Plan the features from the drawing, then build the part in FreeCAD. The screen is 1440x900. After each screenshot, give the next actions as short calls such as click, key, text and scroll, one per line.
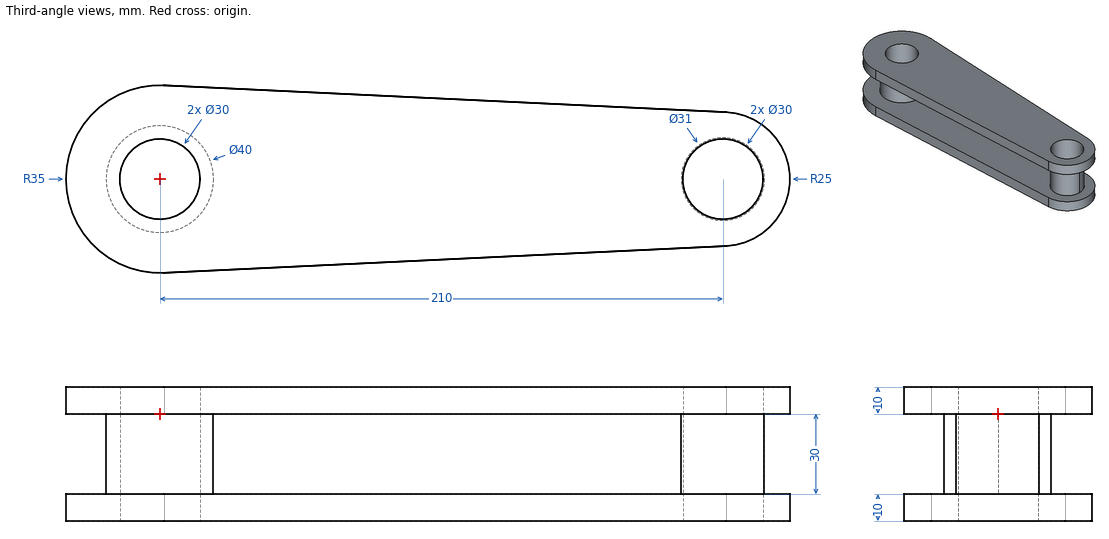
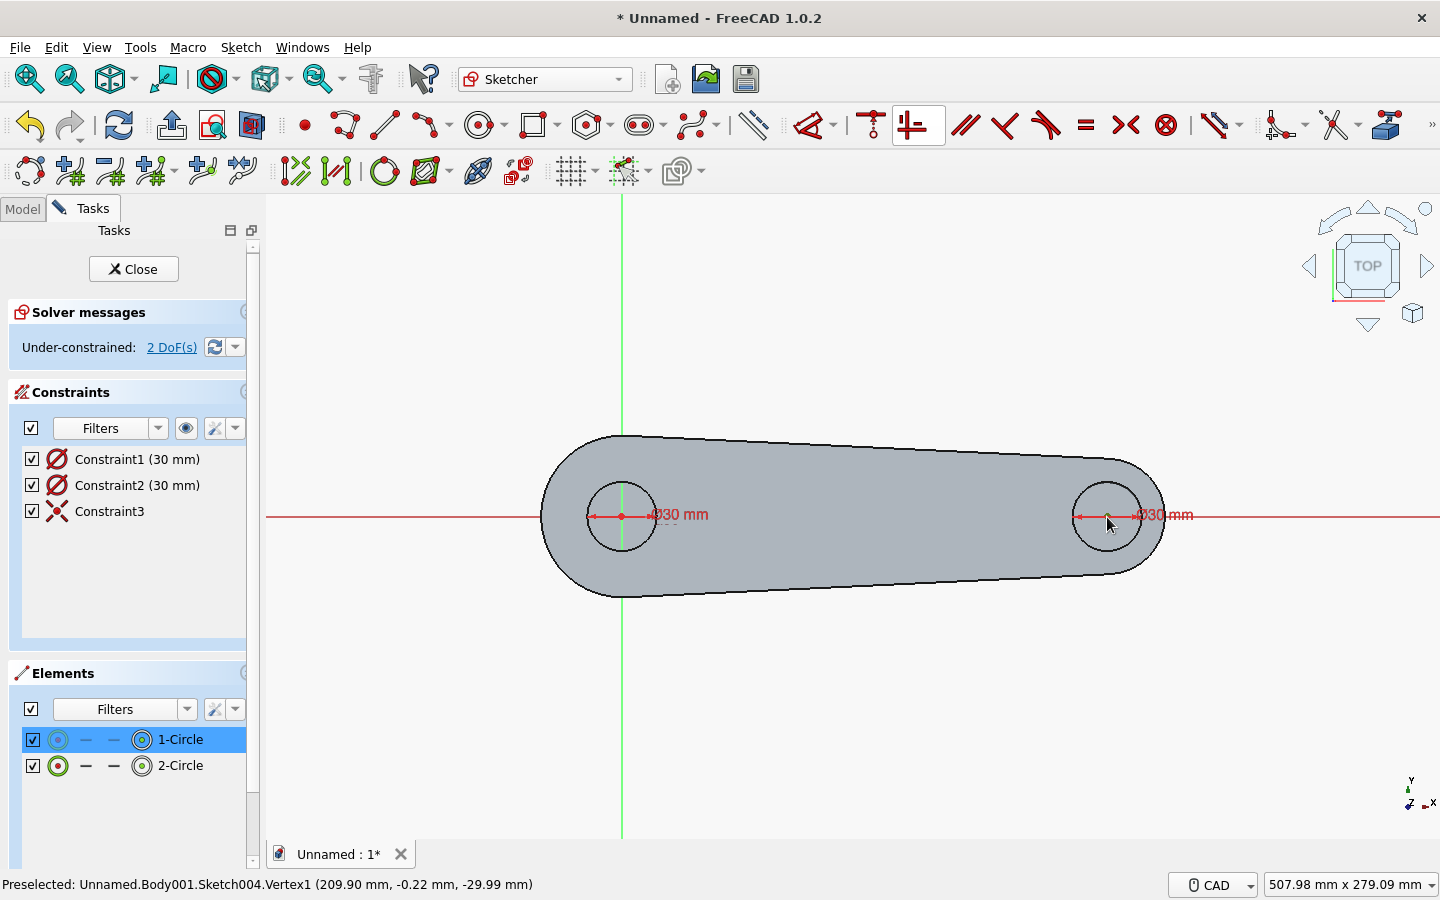
click(364, 516)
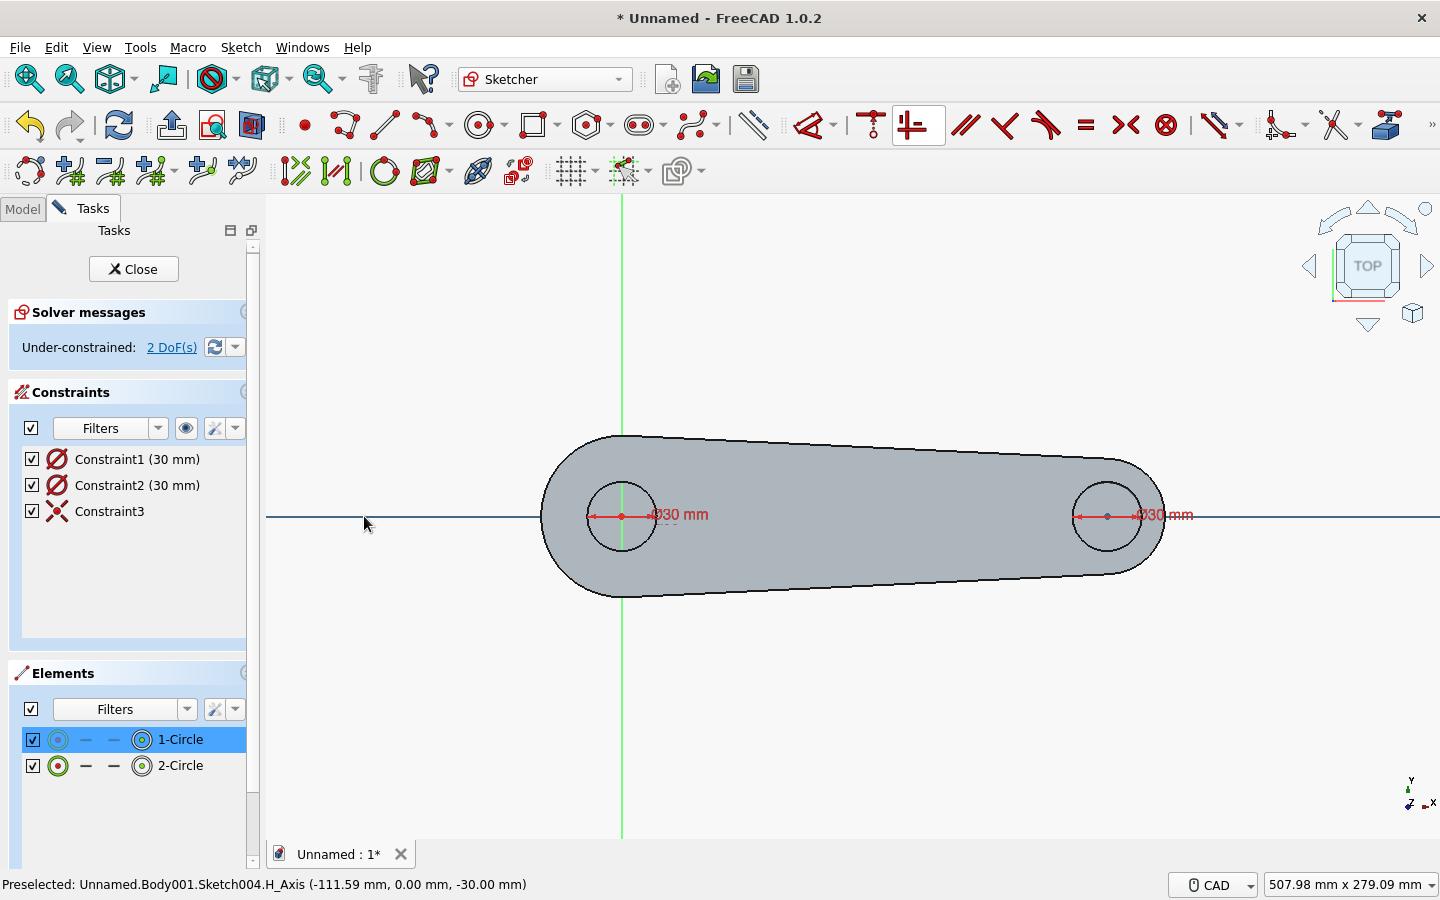
click(872, 126)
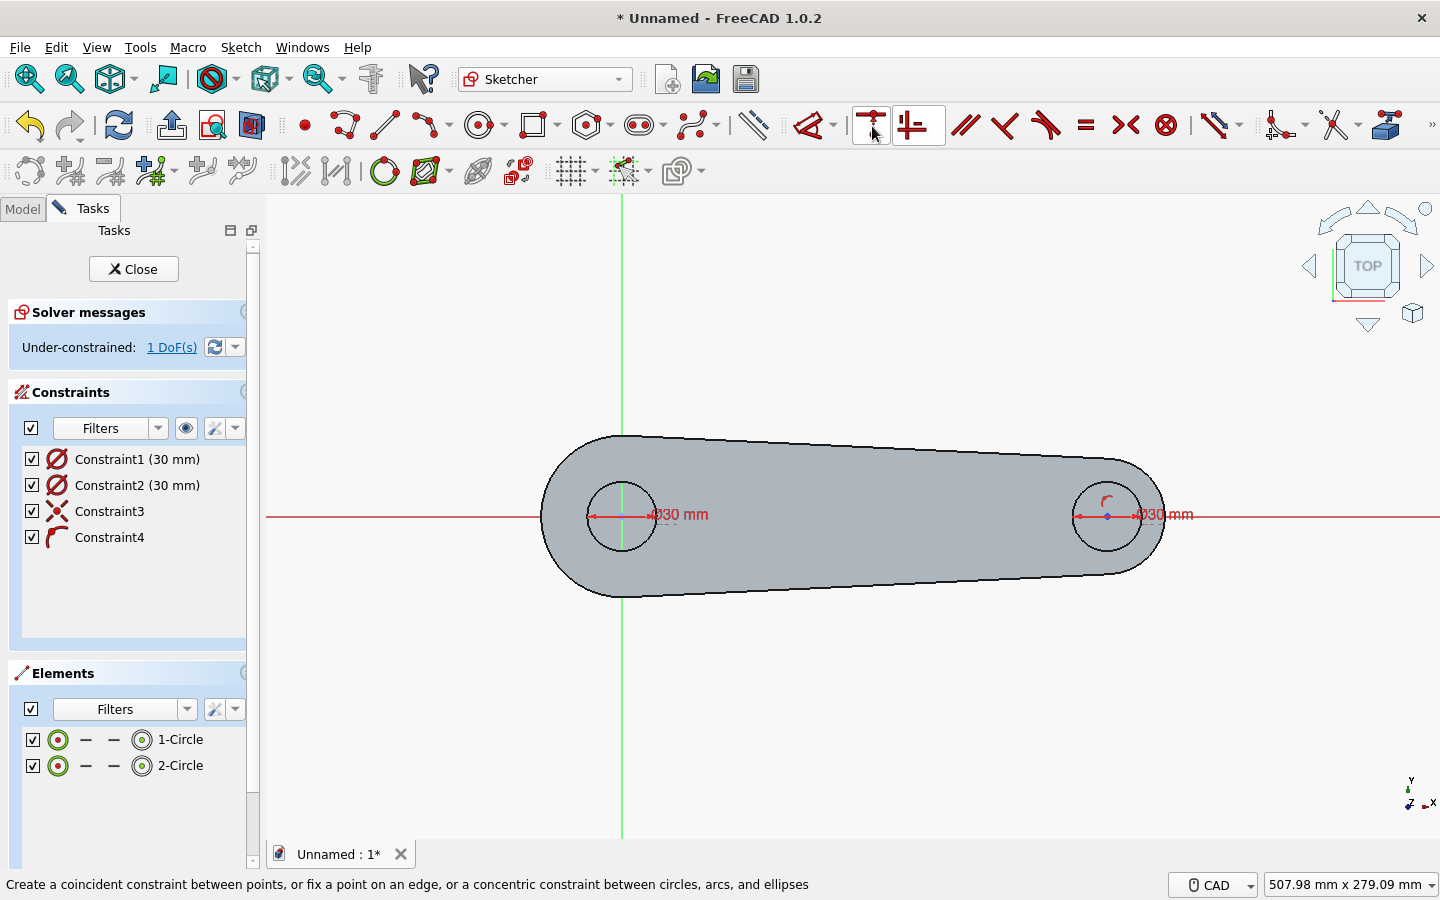
click(808, 126)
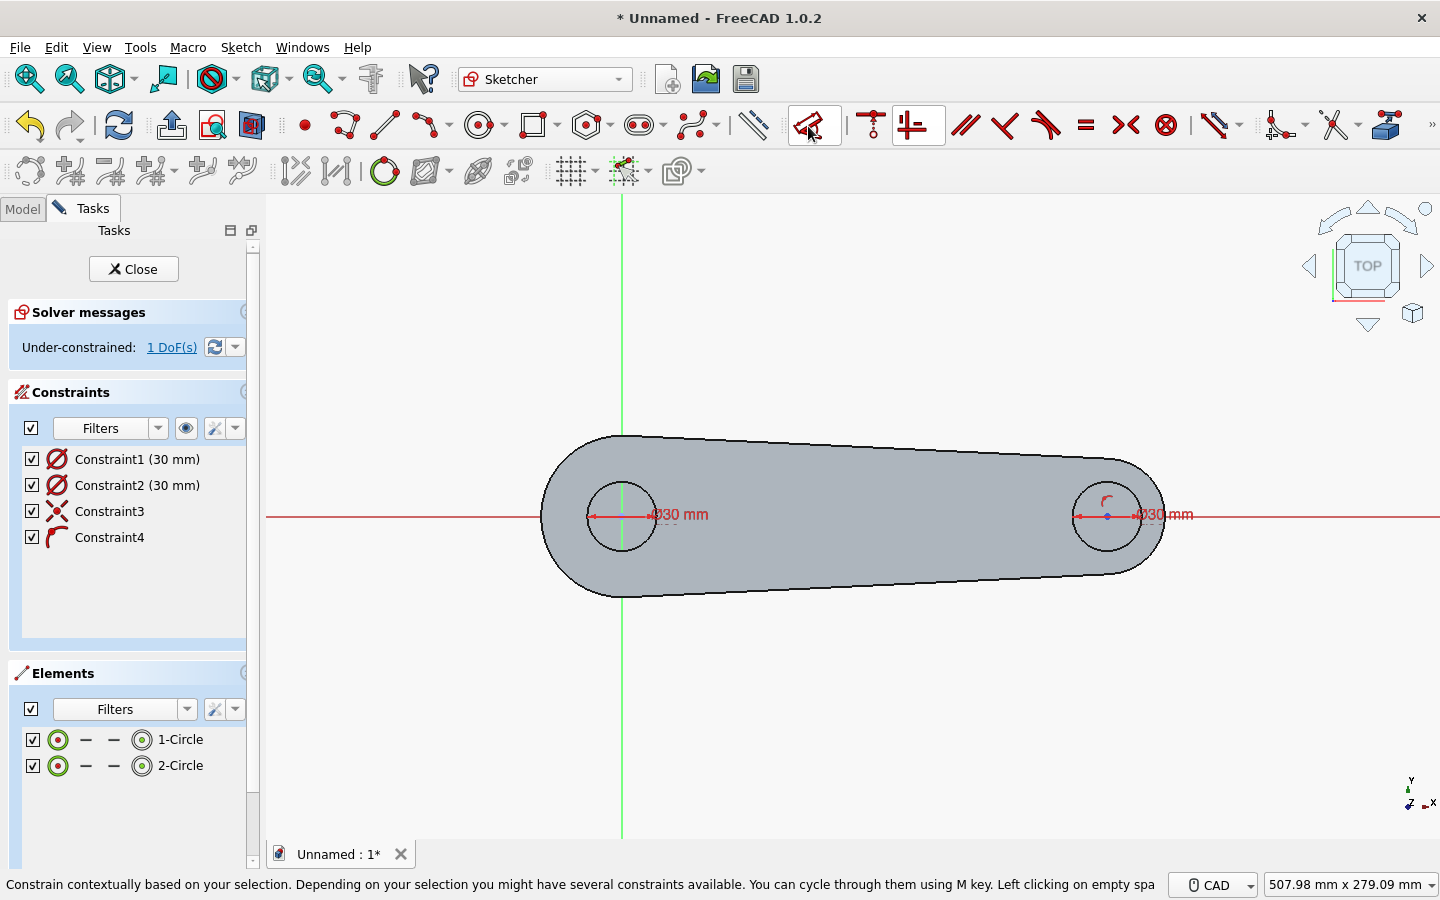
click(1107, 516)
click(864, 550)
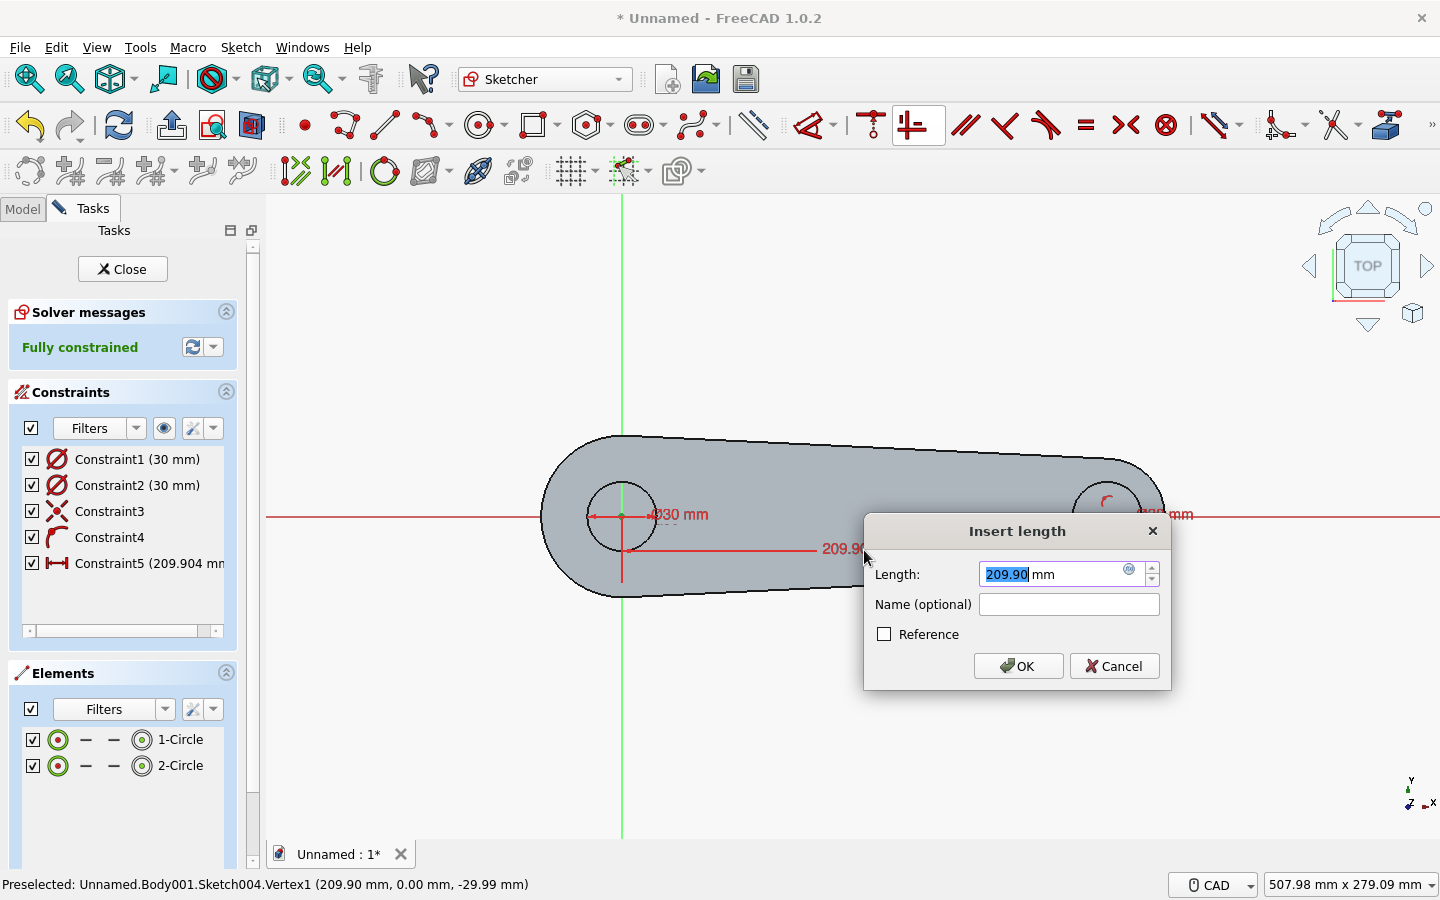
text(210)
key(Return)
key(Escape)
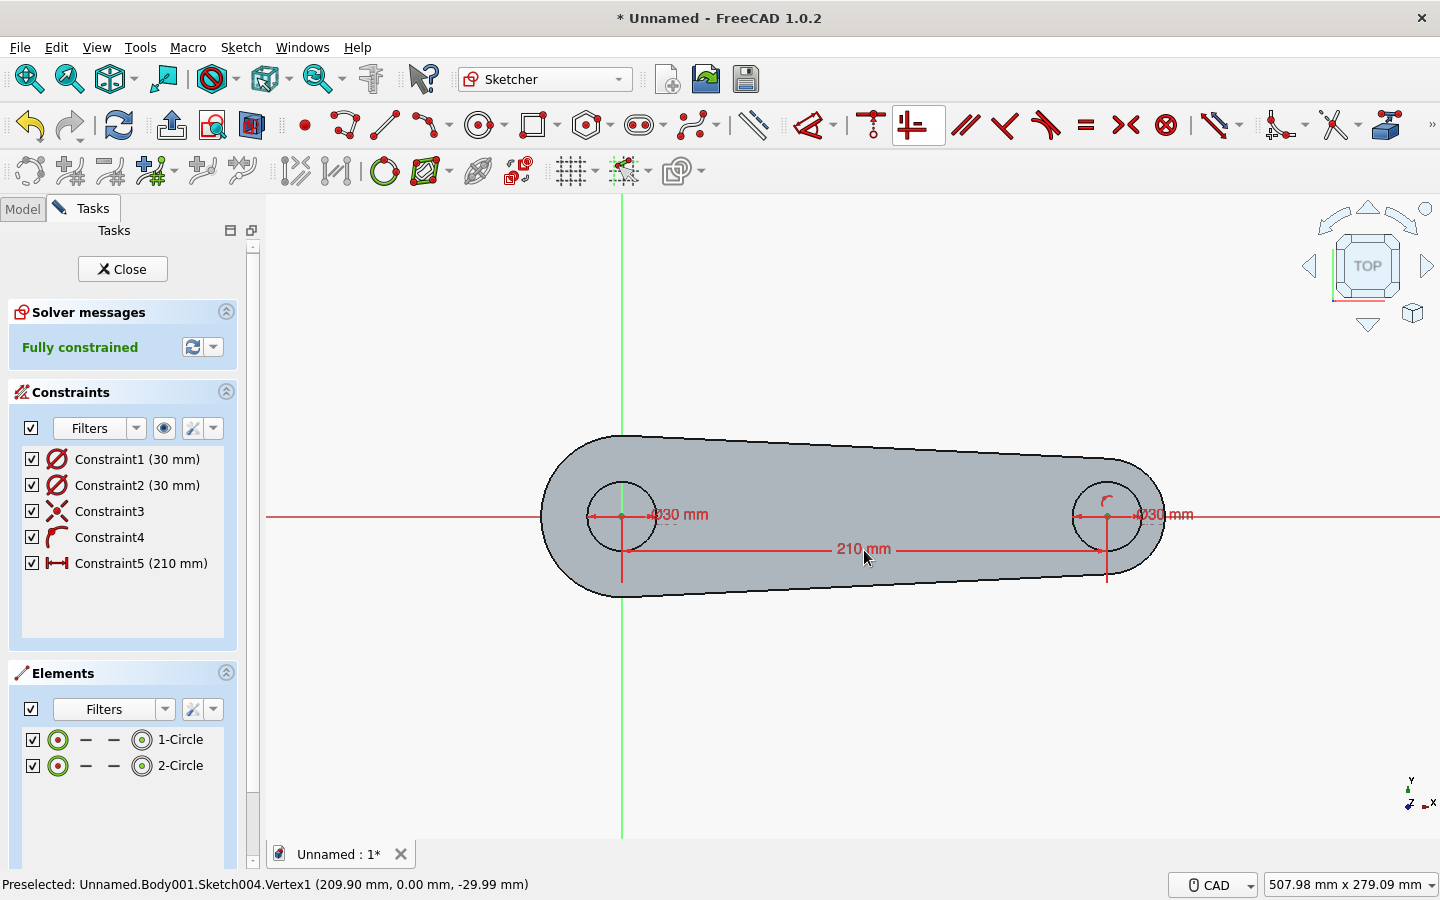
click(123, 269)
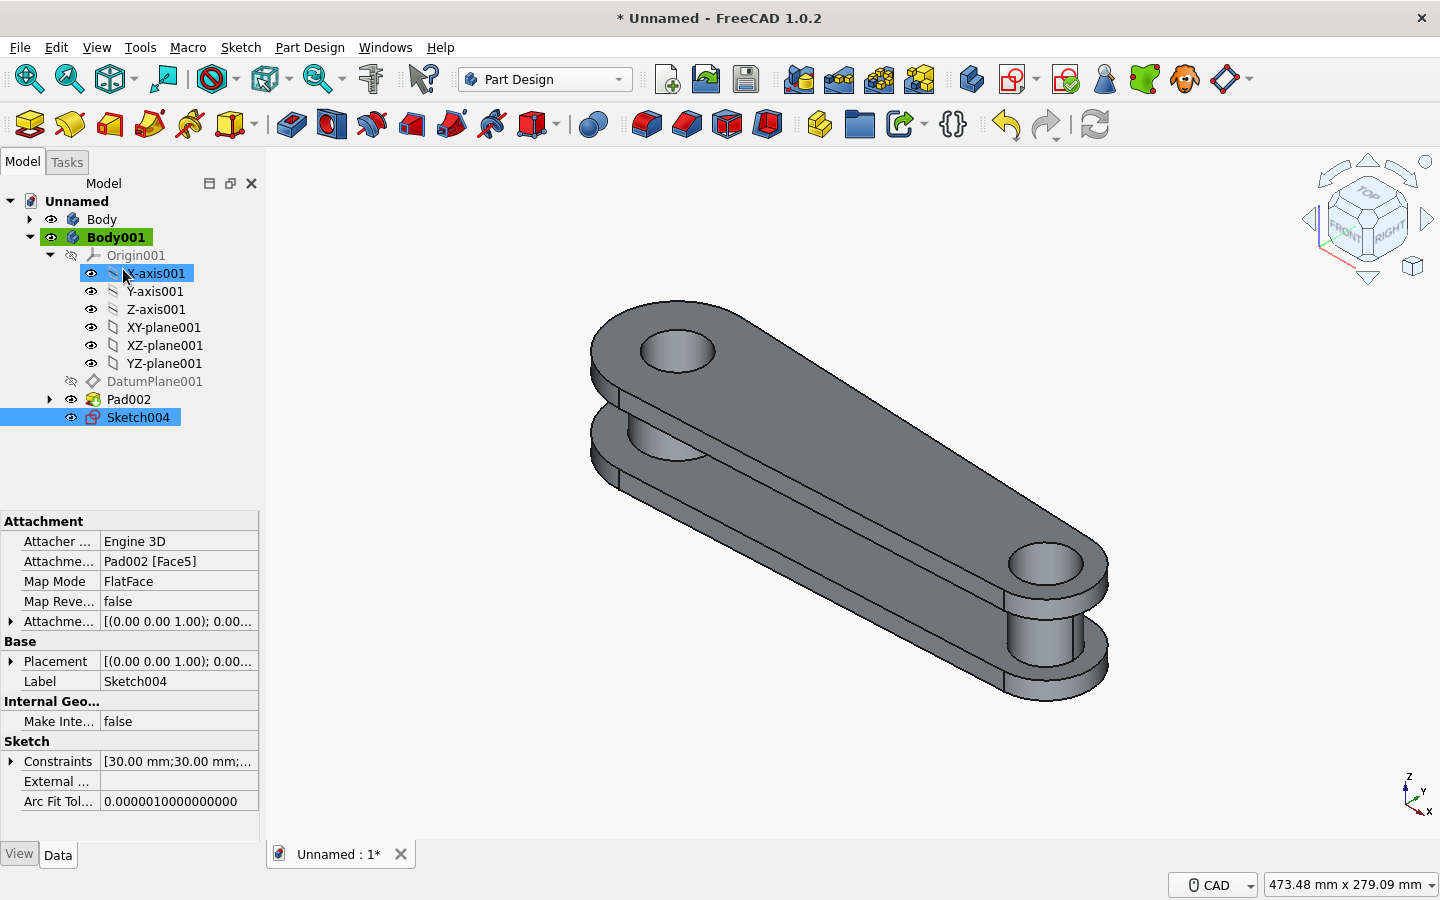
click(292, 124)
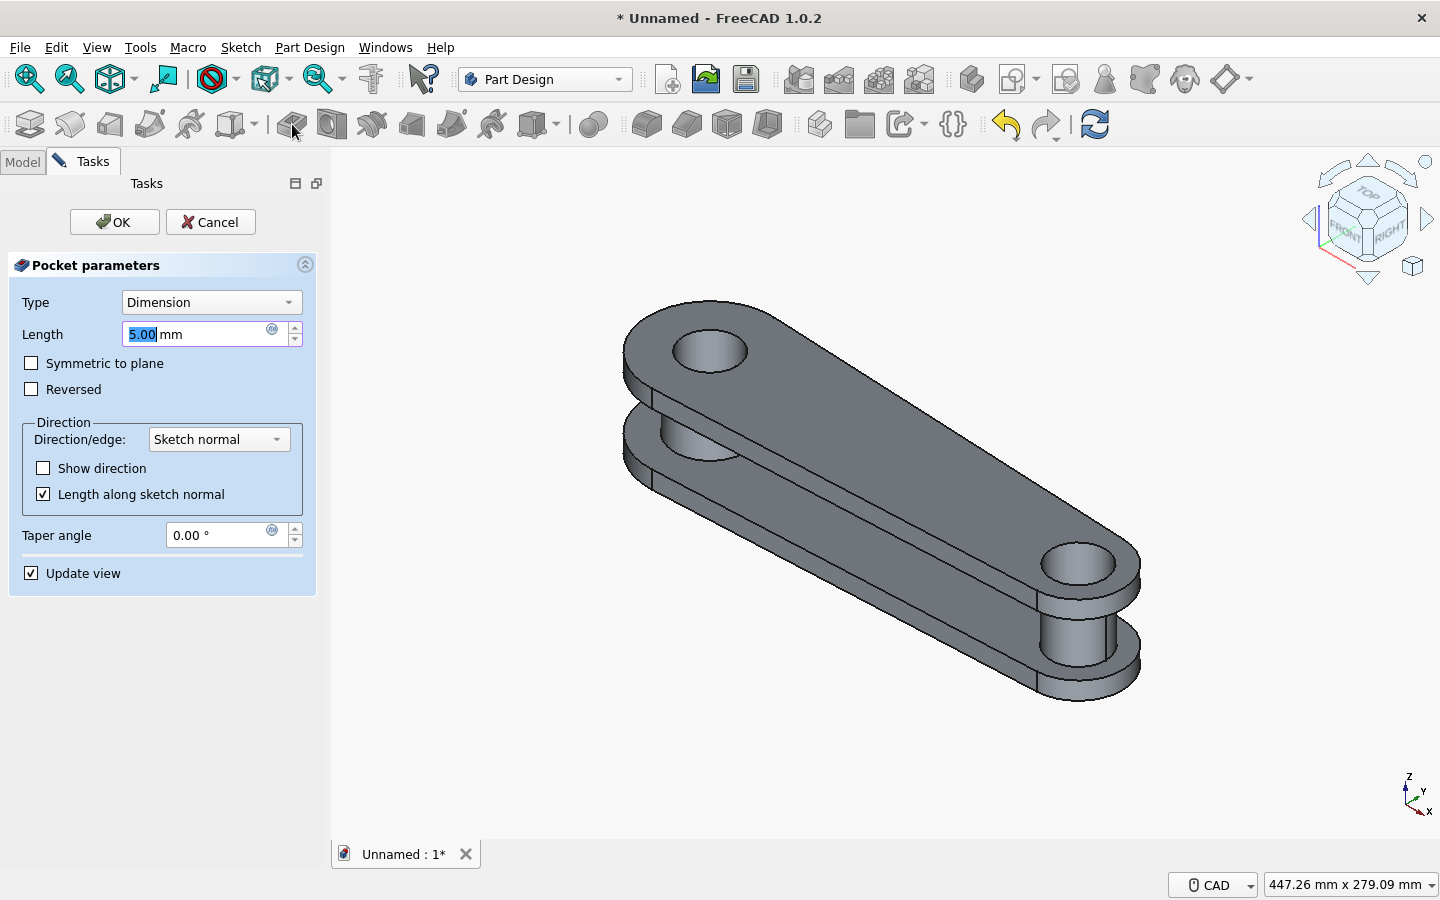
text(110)
key(Tab)